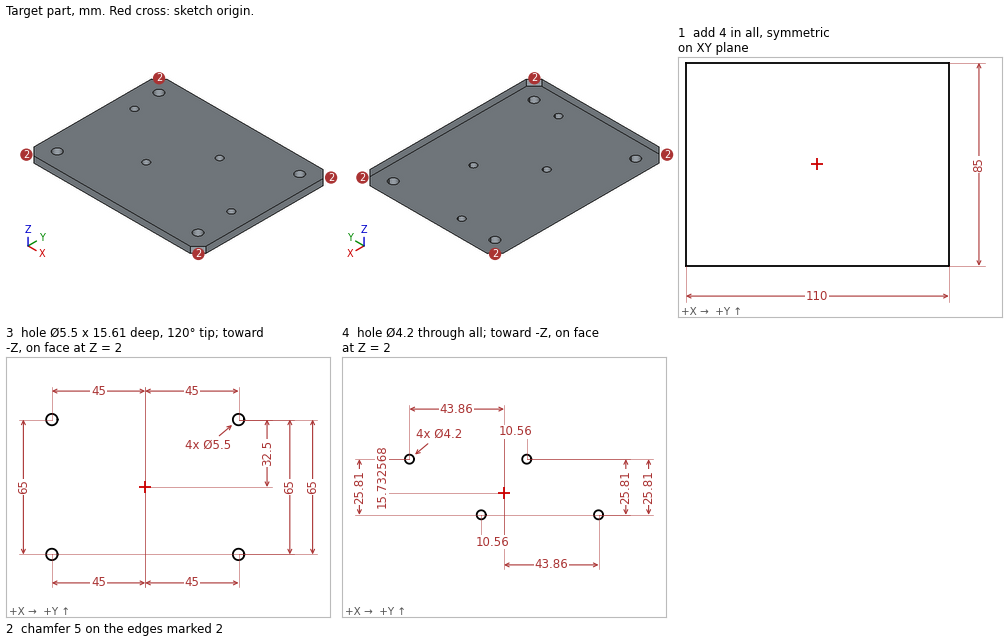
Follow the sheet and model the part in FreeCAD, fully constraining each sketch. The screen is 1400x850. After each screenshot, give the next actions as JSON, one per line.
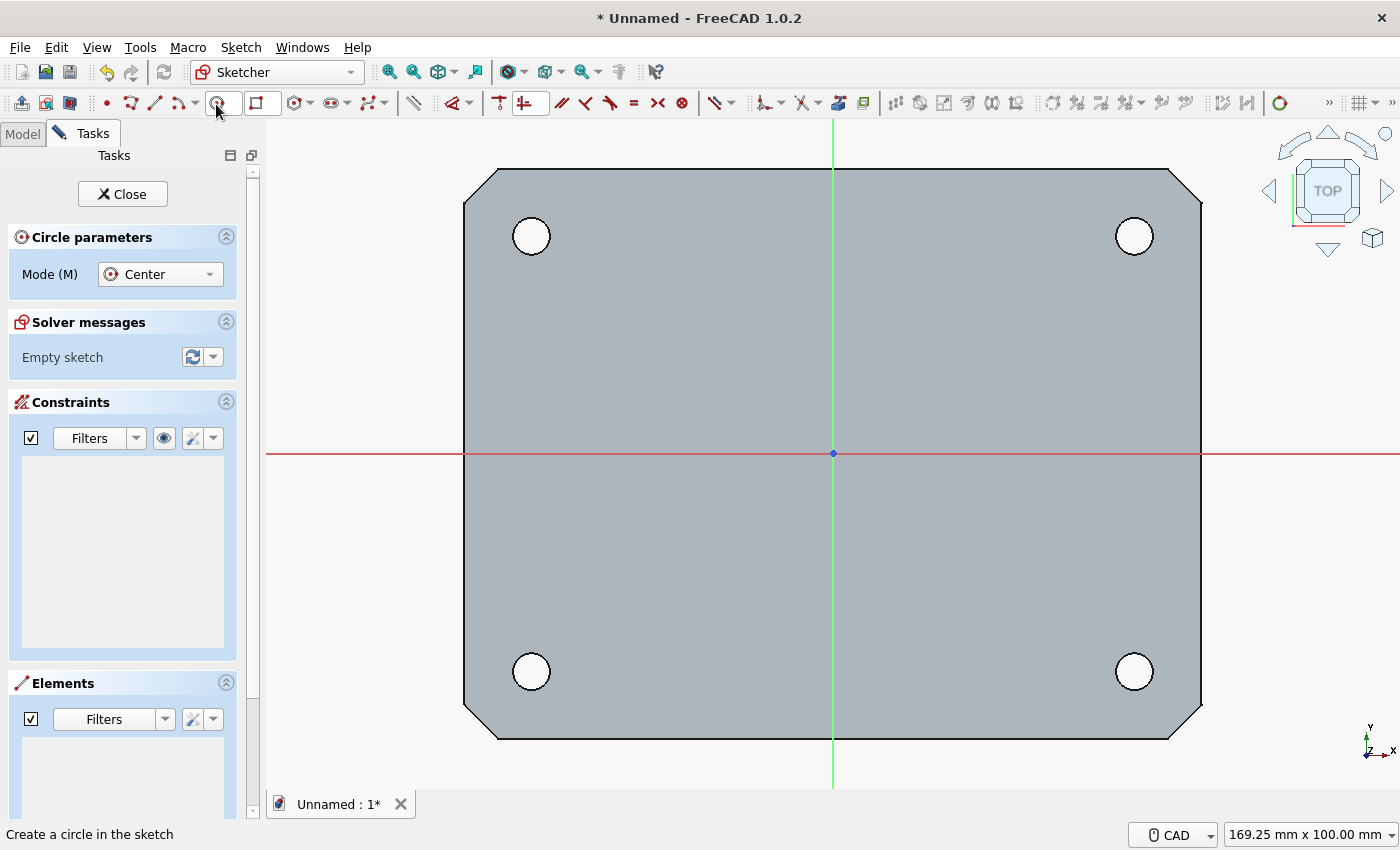
{"action": "scroll", "coordinate": [539, 349], "scroll_direction": "up", "scroll_amount": 3}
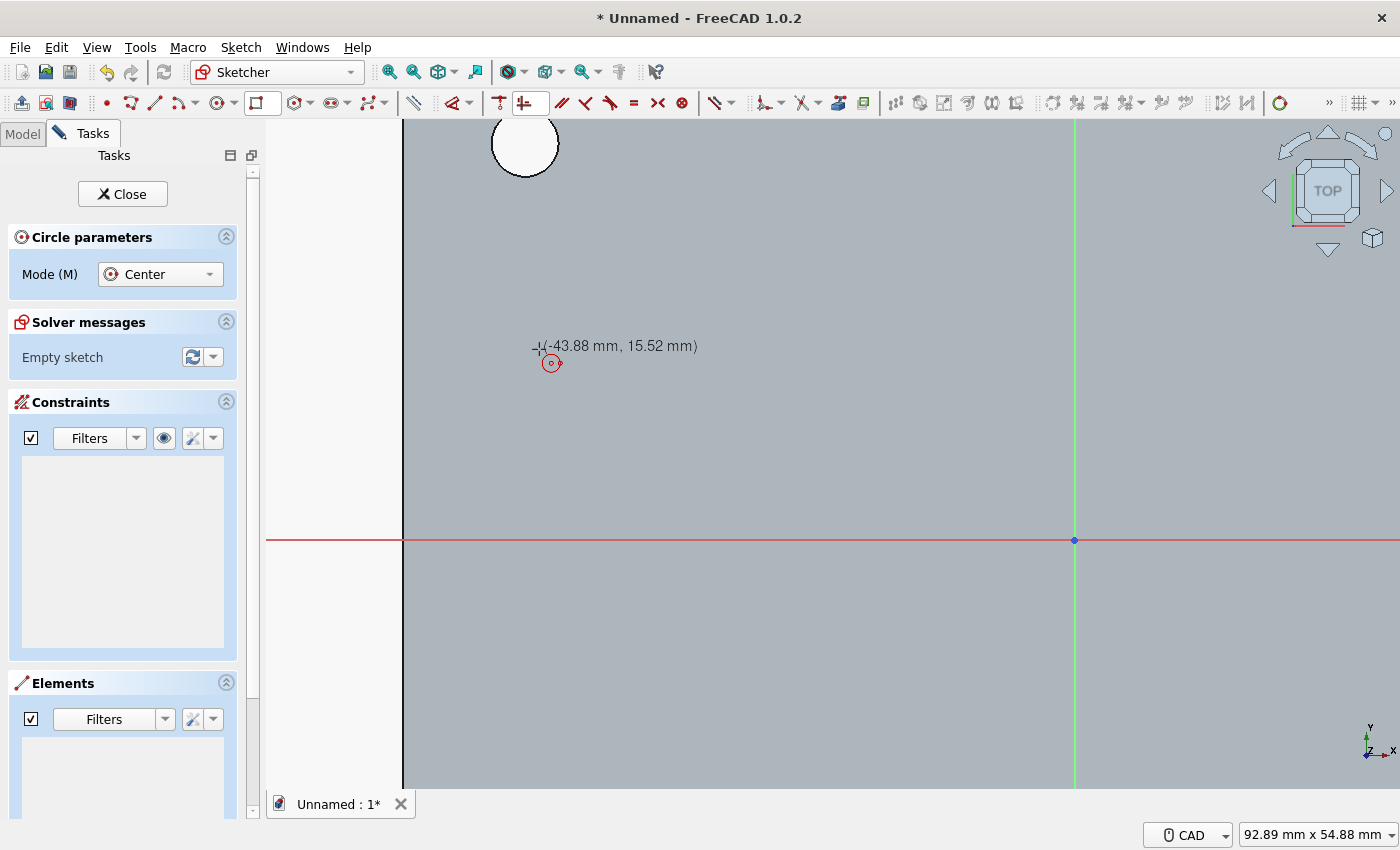
{"action": "left_click", "coordinate": [539, 348]}
{"action": "mouse_move", "coordinate": [557, 330]}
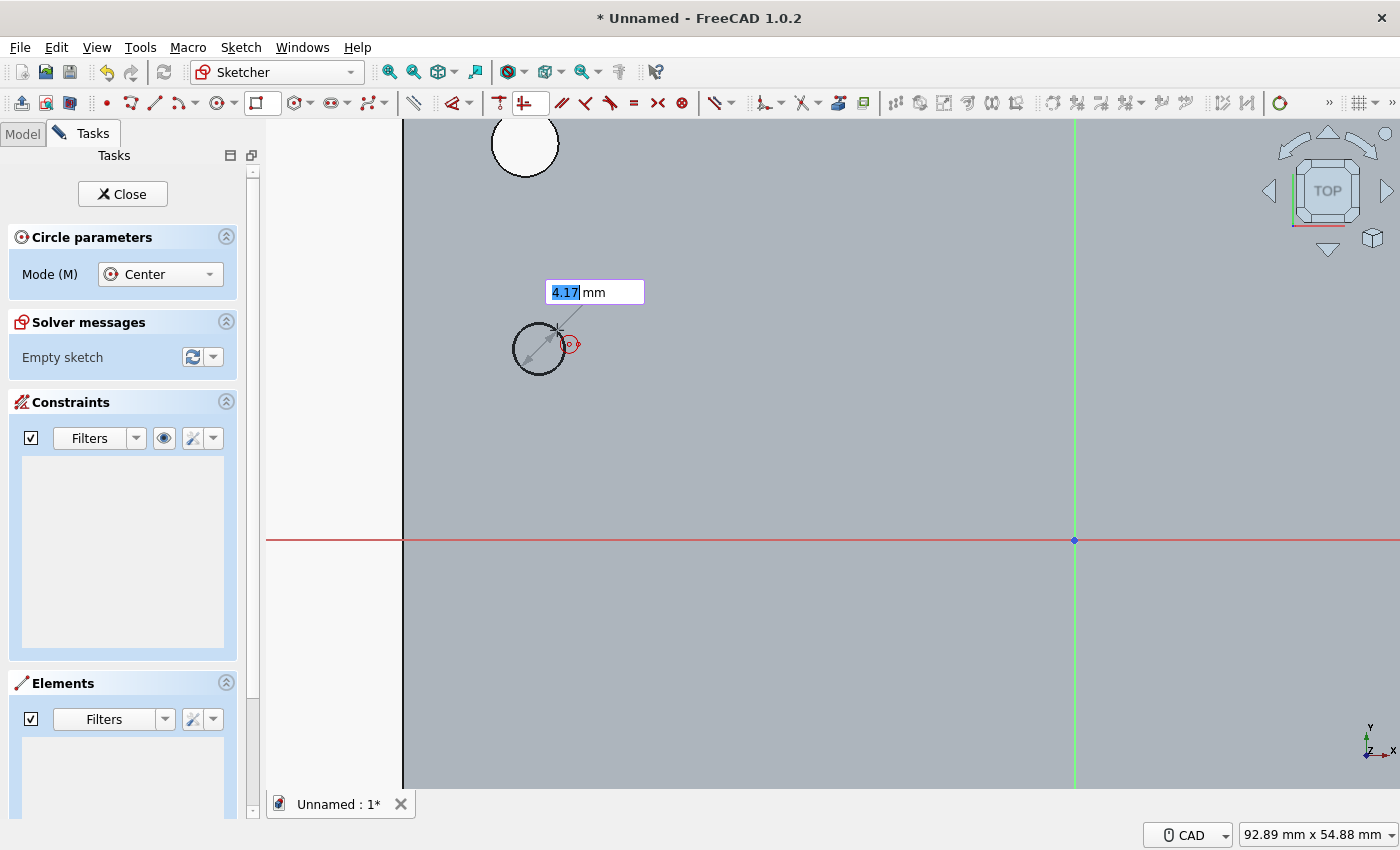
{"action": "type", "text": "4.2"}
{"action": "key", "text": "Return"}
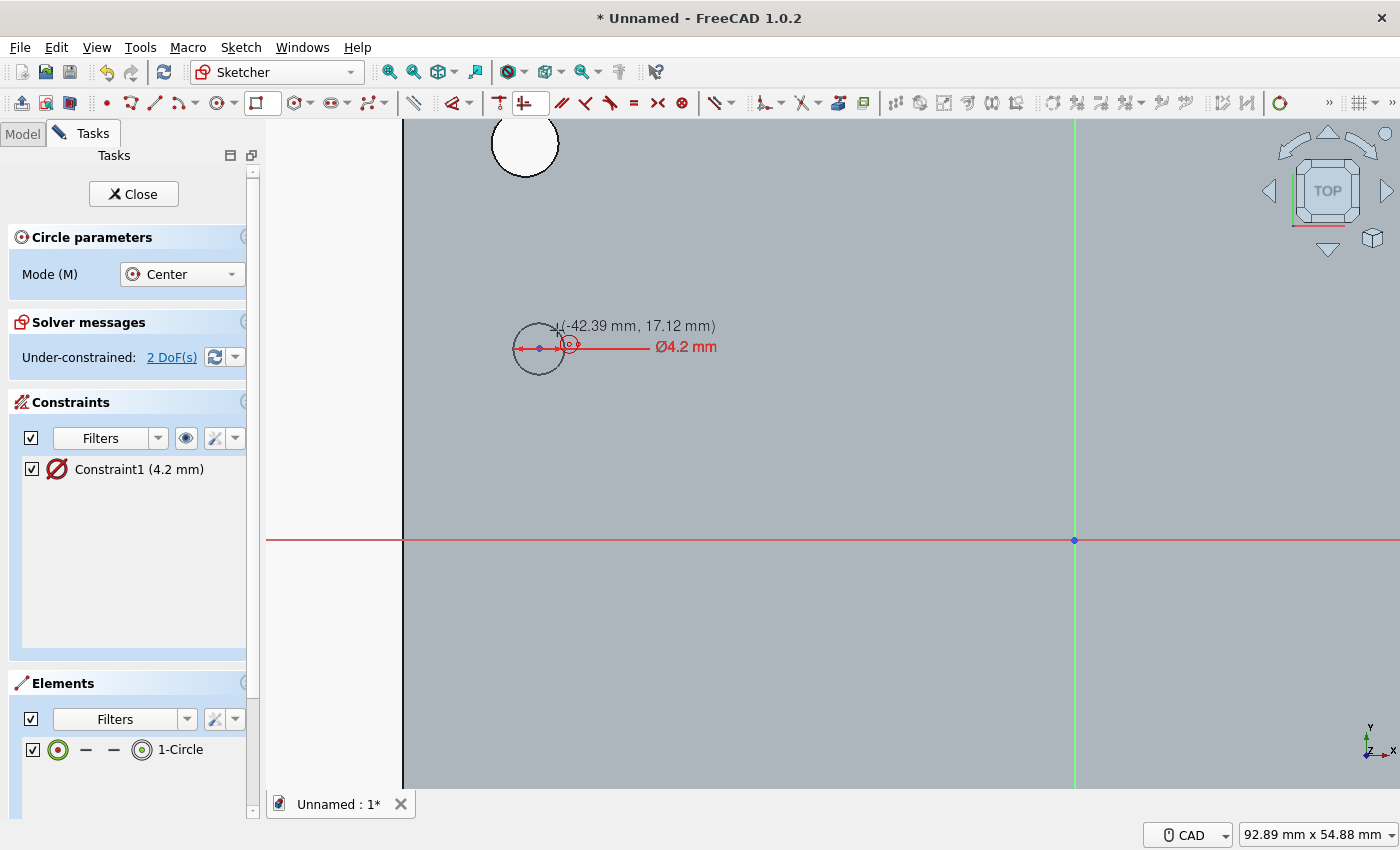
{"action": "left_click", "coordinate": [1203, 348]}
{"action": "mouse_move", "coordinate": [1222, 330]}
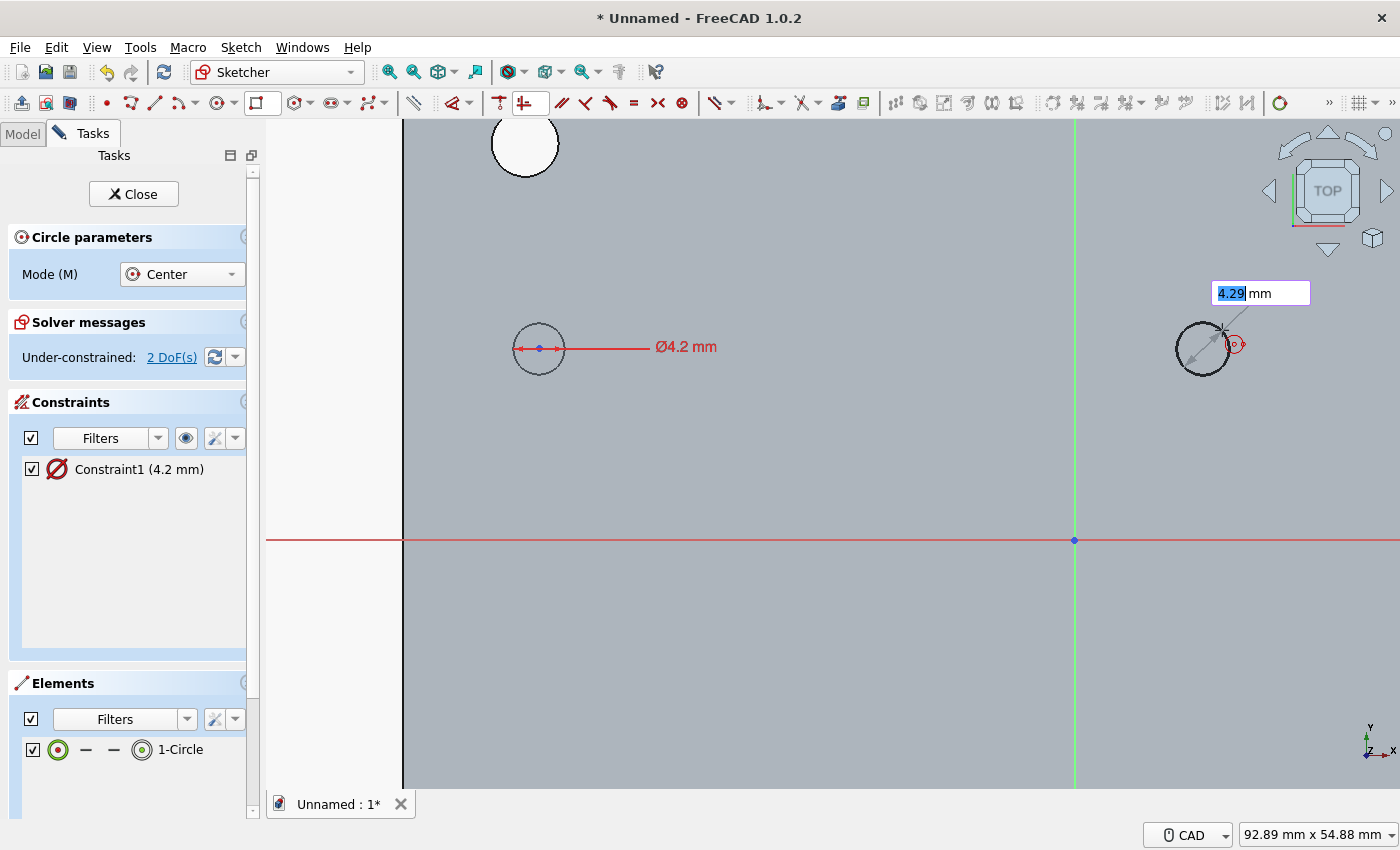
{"action": "type", "text": "4.2"}
{"action": "key", "text": "Return"}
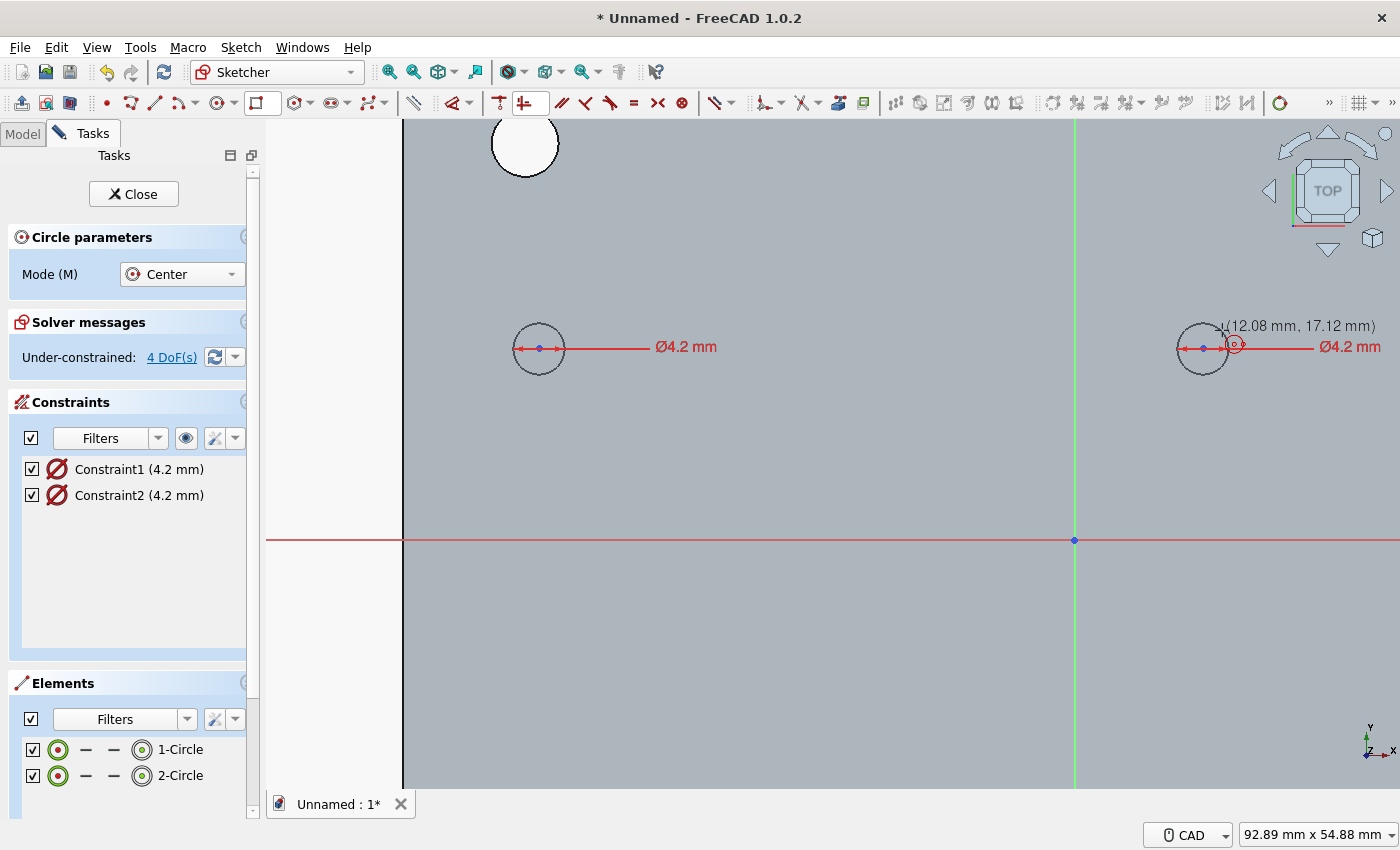
{"action": "left_click", "coordinate": [946, 663]}
{"action": "mouse_move", "coordinate": [964, 645]}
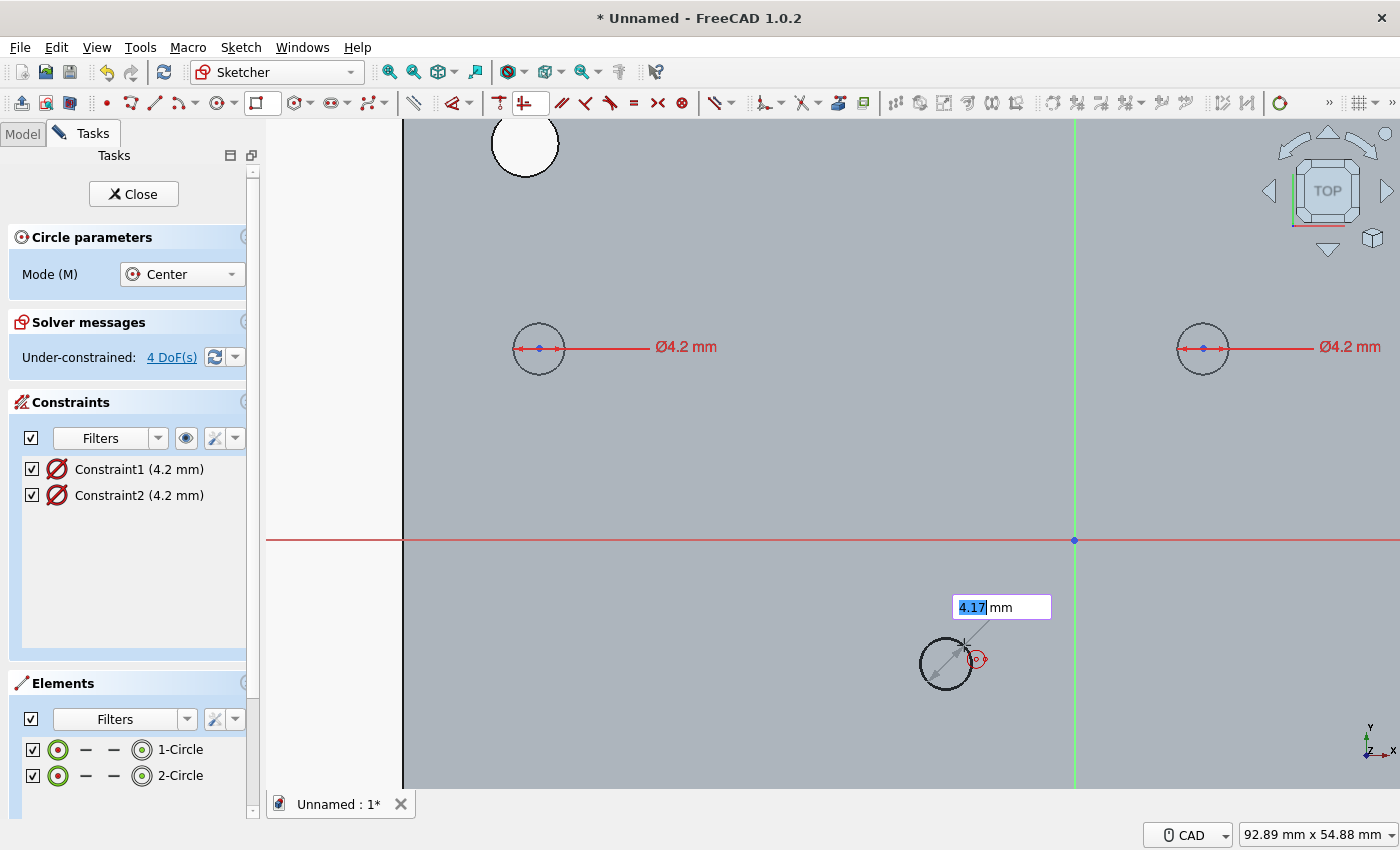
{"action": "type", "text": "4.2"}
{"action": "key", "text": "Return"}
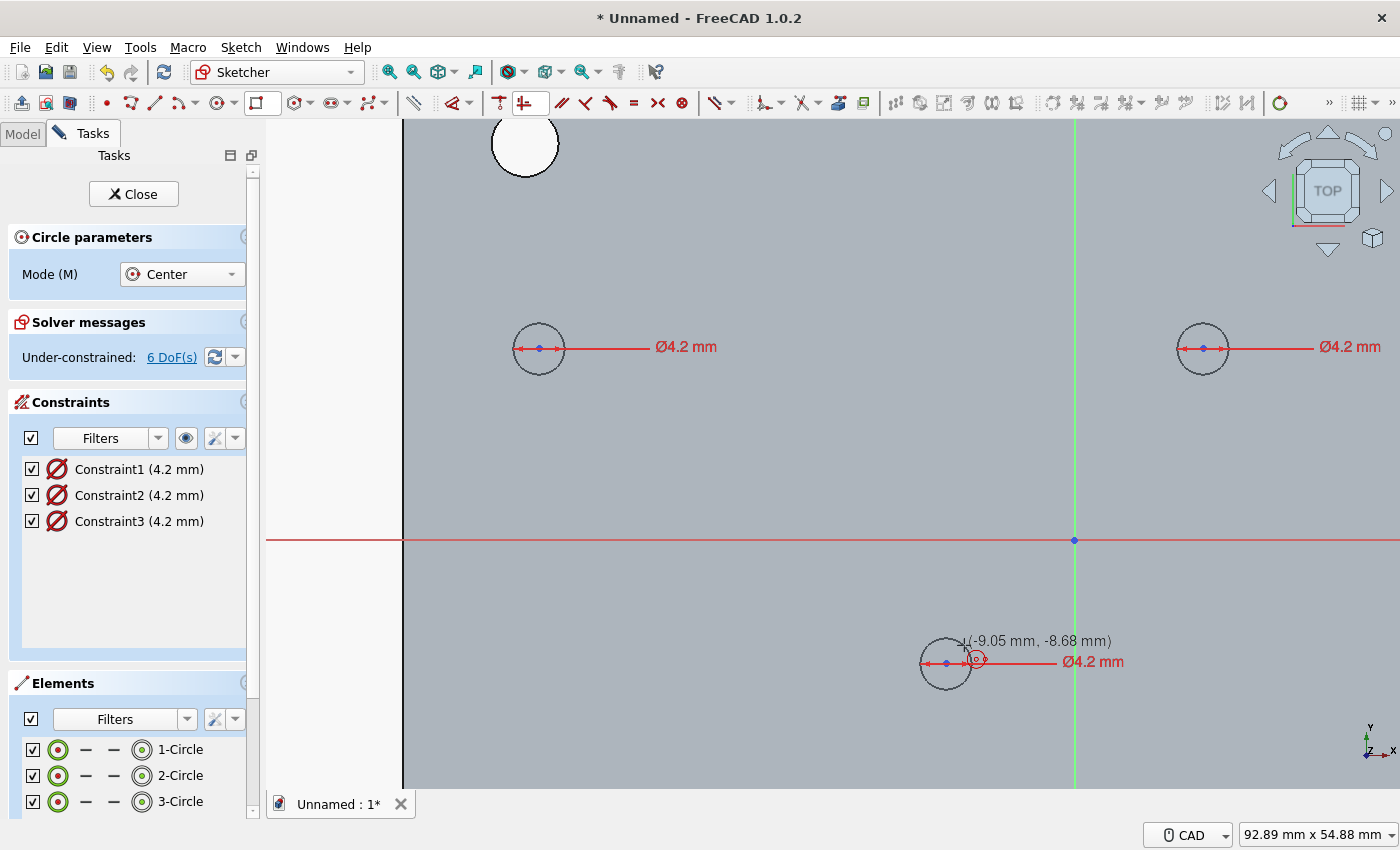
{"action": "scroll", "coordinate": [387, 391], "scroll_direction": "down", "scroll_amount": 3}